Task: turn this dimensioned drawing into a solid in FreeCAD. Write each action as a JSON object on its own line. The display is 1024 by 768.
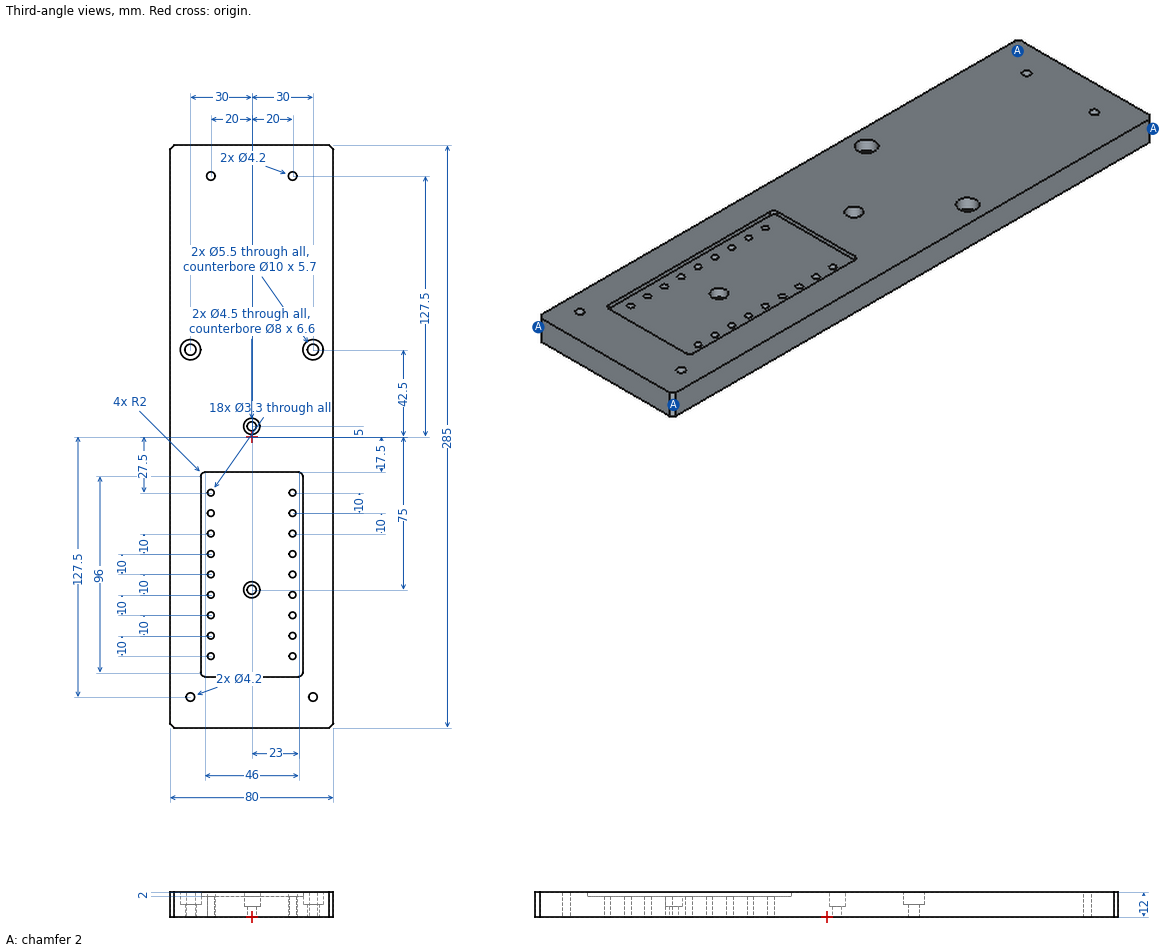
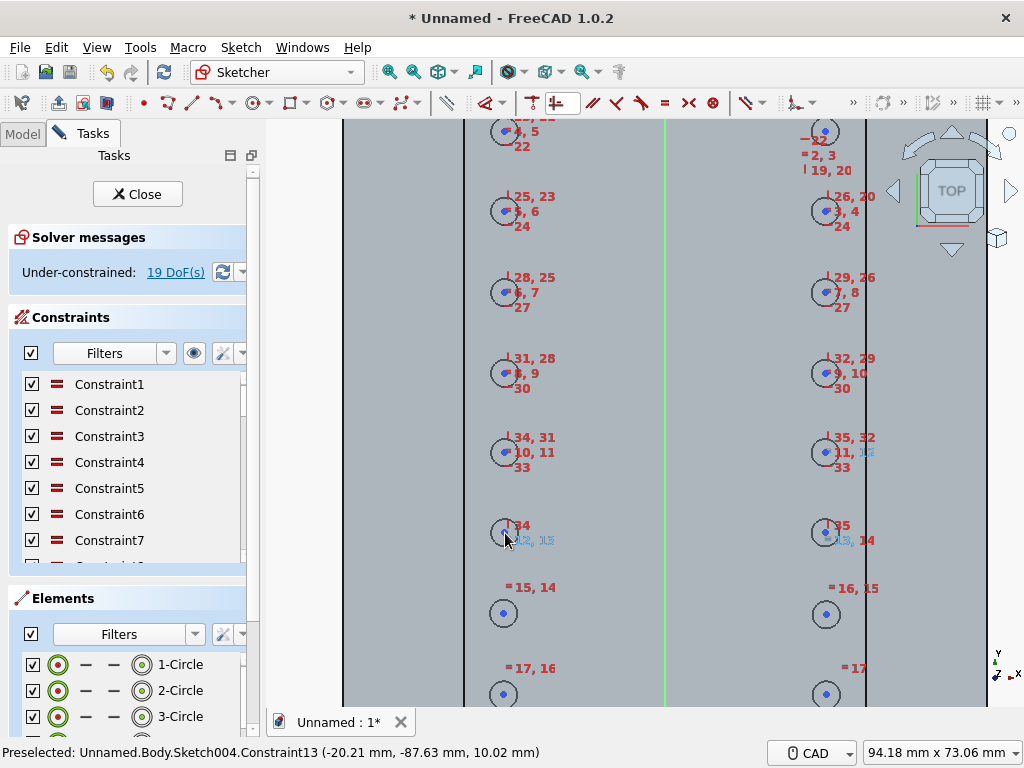
{"action": "scroll", "coordinate": [505, 533], "scroll_direction": "up", "scroll_amount": 4}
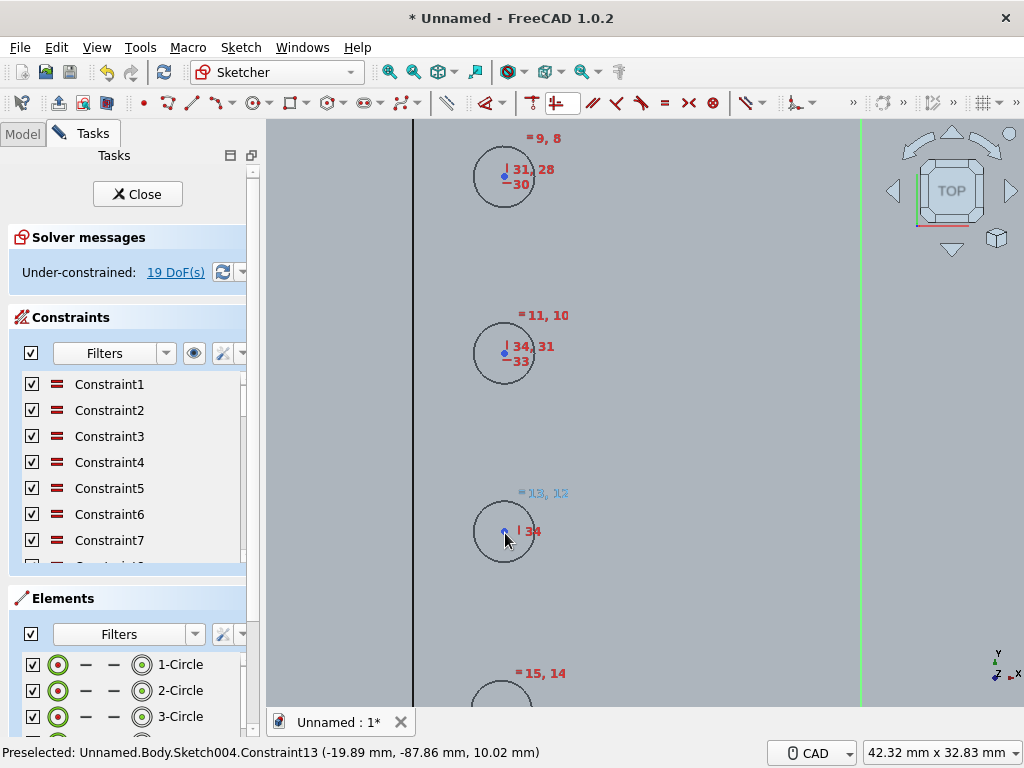
{"action": "left_click", "coordinate": [504, 532]}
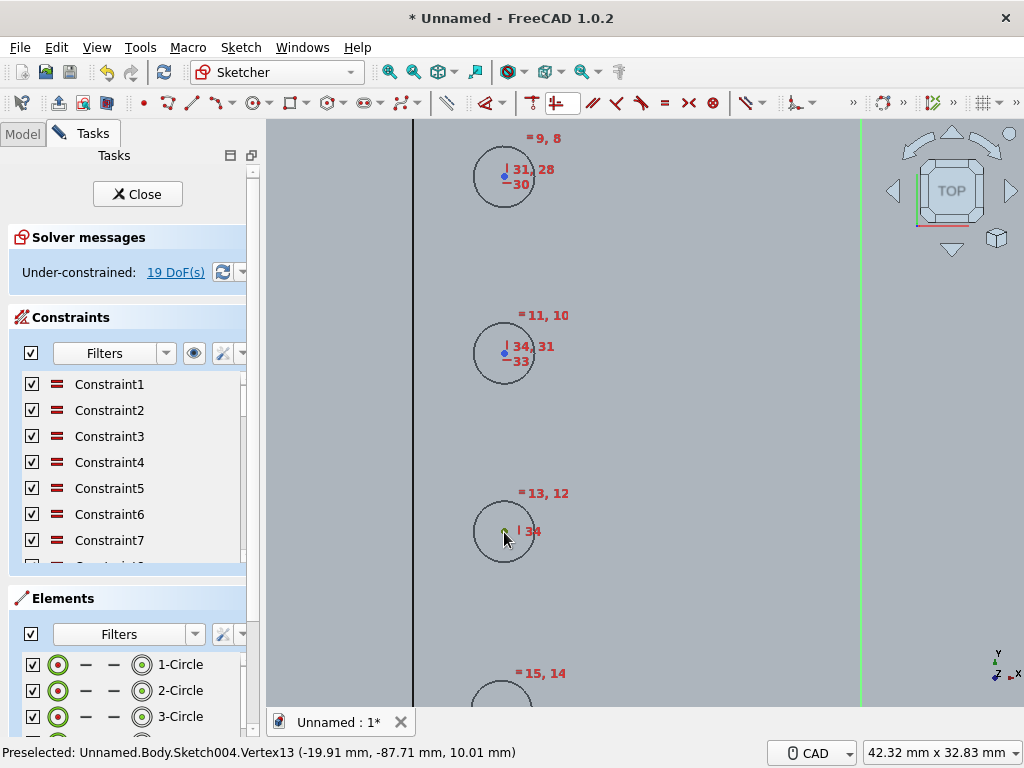
{"action": "scroll", "coordinate": [505, 533], "scroll_direction": "down", "scroll_amount": 8}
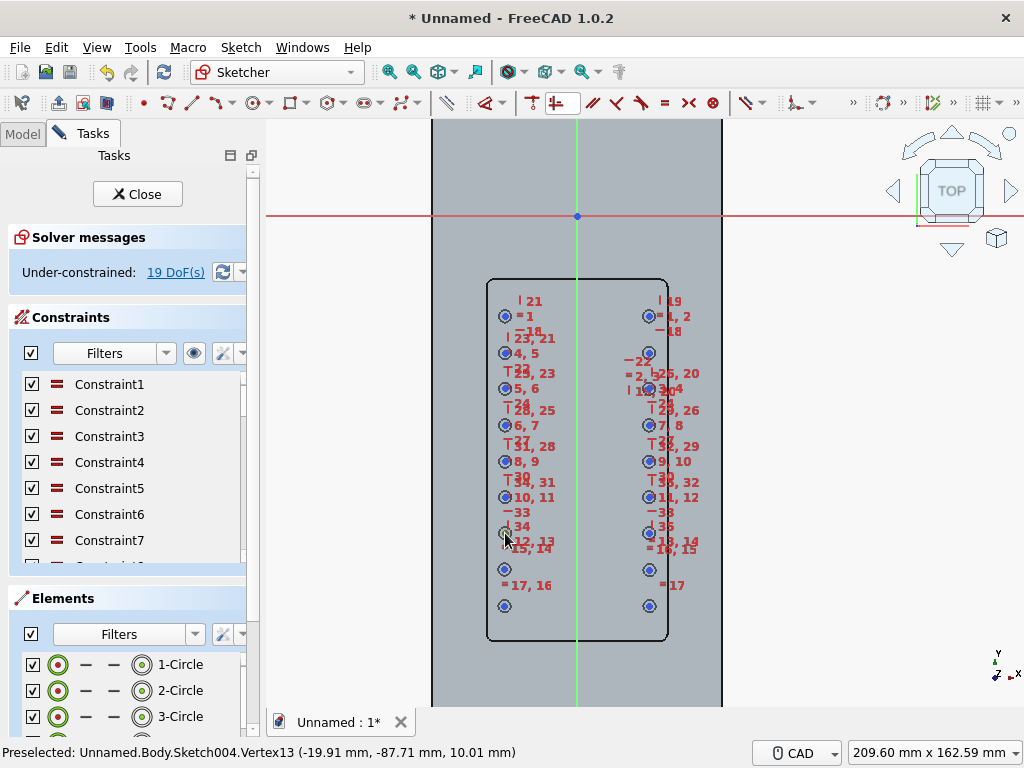
{"action": "scroll", "coordinate": [649, 533], "scroll_direction": "up", "scroll_amount": 4}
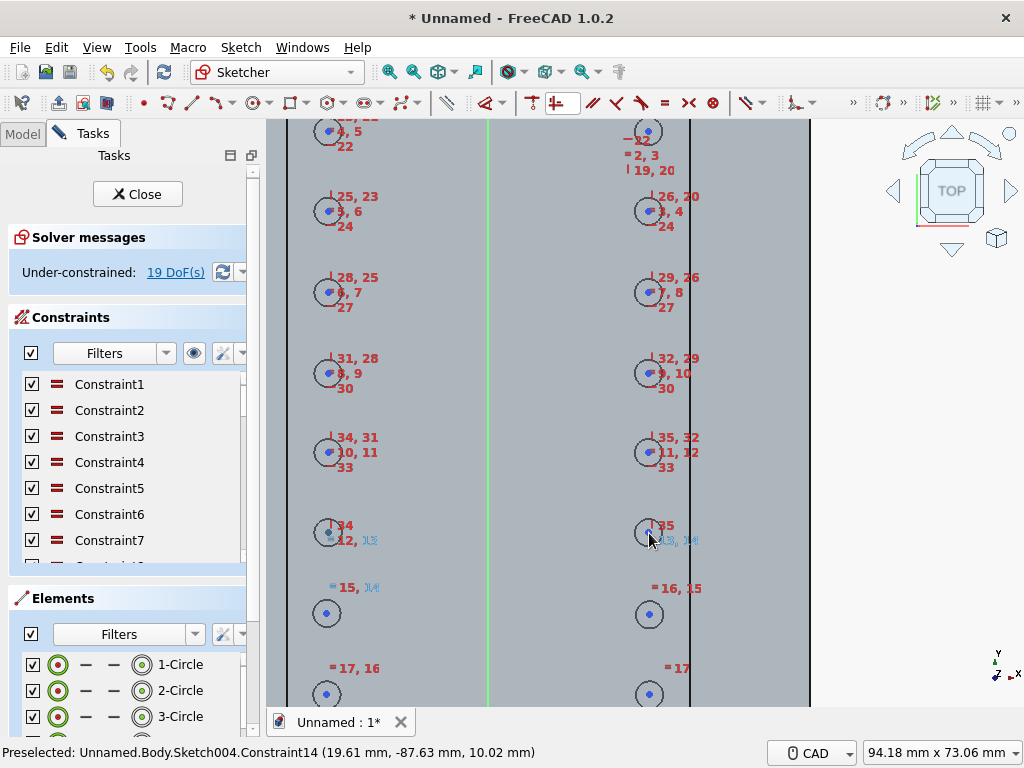
{"action": "scroll", "coordinate": [649, 533], "scroll_direction": "up", "scroll_amount": 4}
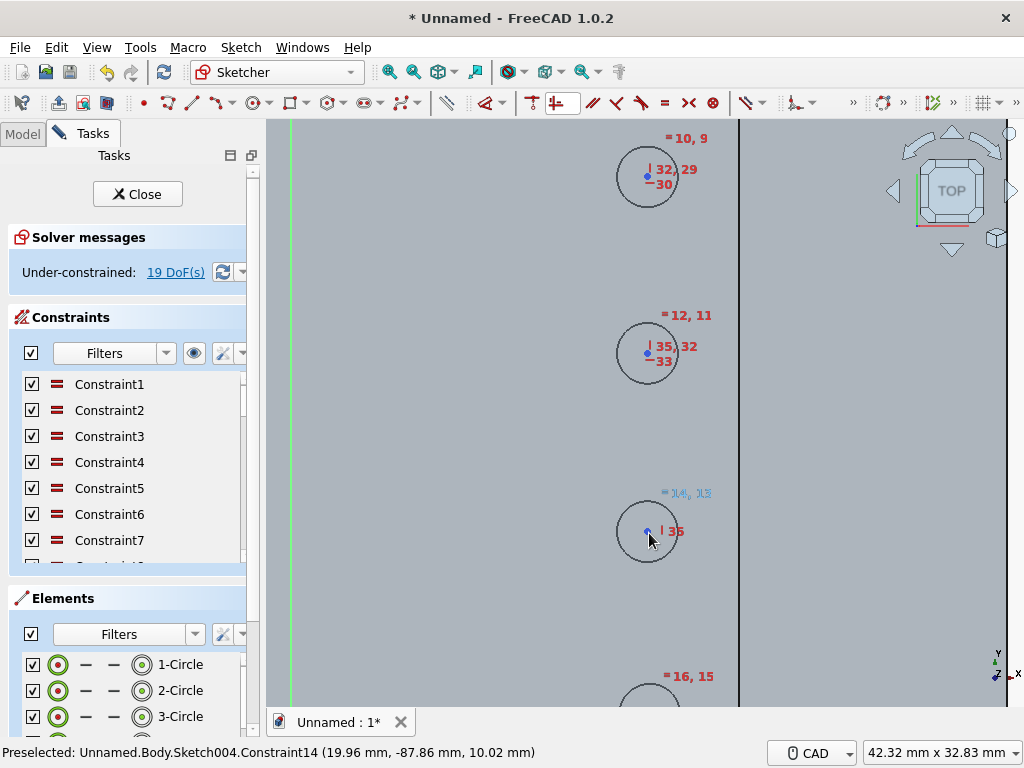
{"action": "left_click", "coordinate": [647, 532]}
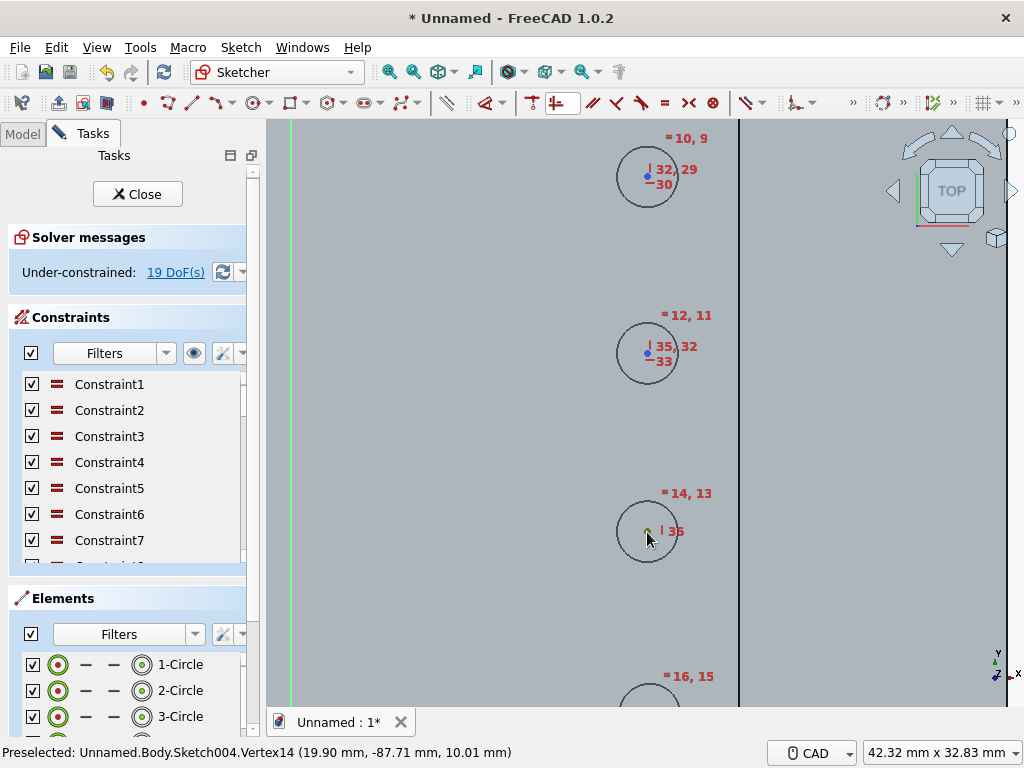
{"action": "key", "text": "h"}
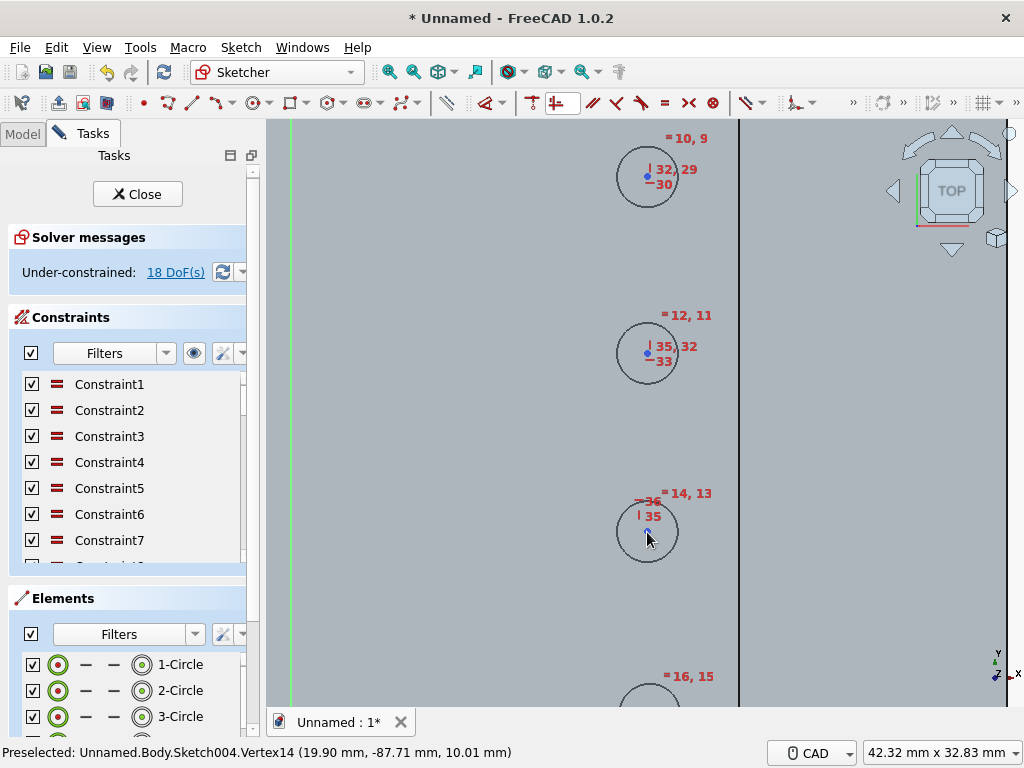
{"action": "scroll", "coordinate": [649, 533], "scroll_direction": "down", "scroll_amount": 8}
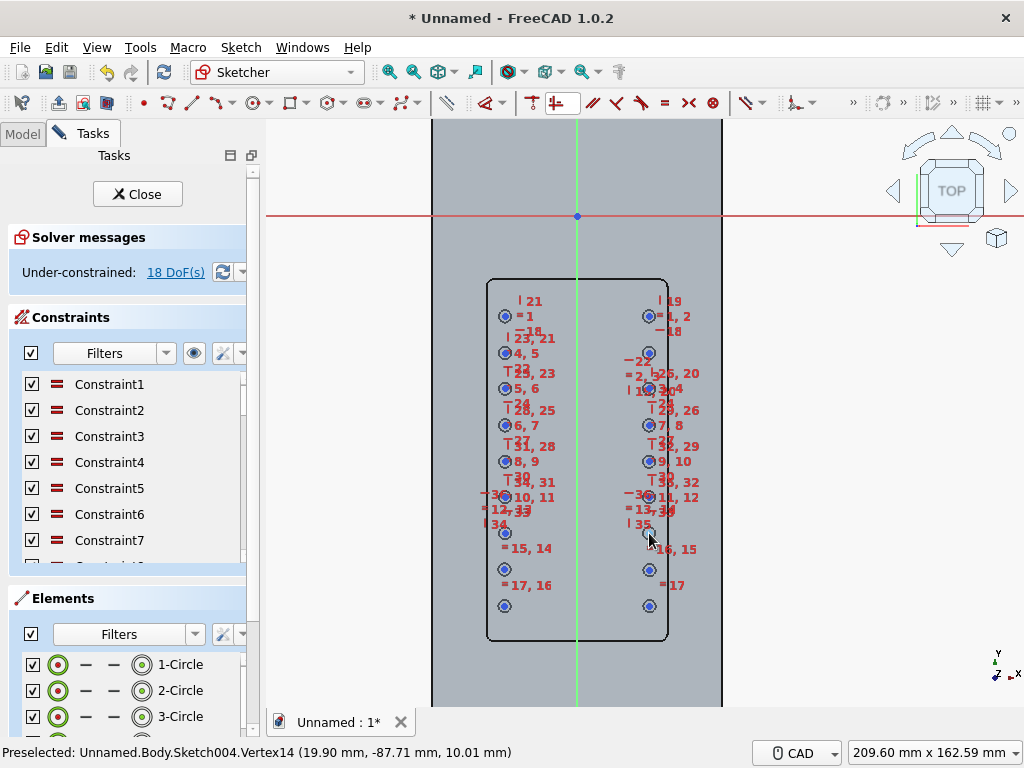
{"action": "left_click", "coordinate": [505, 533]}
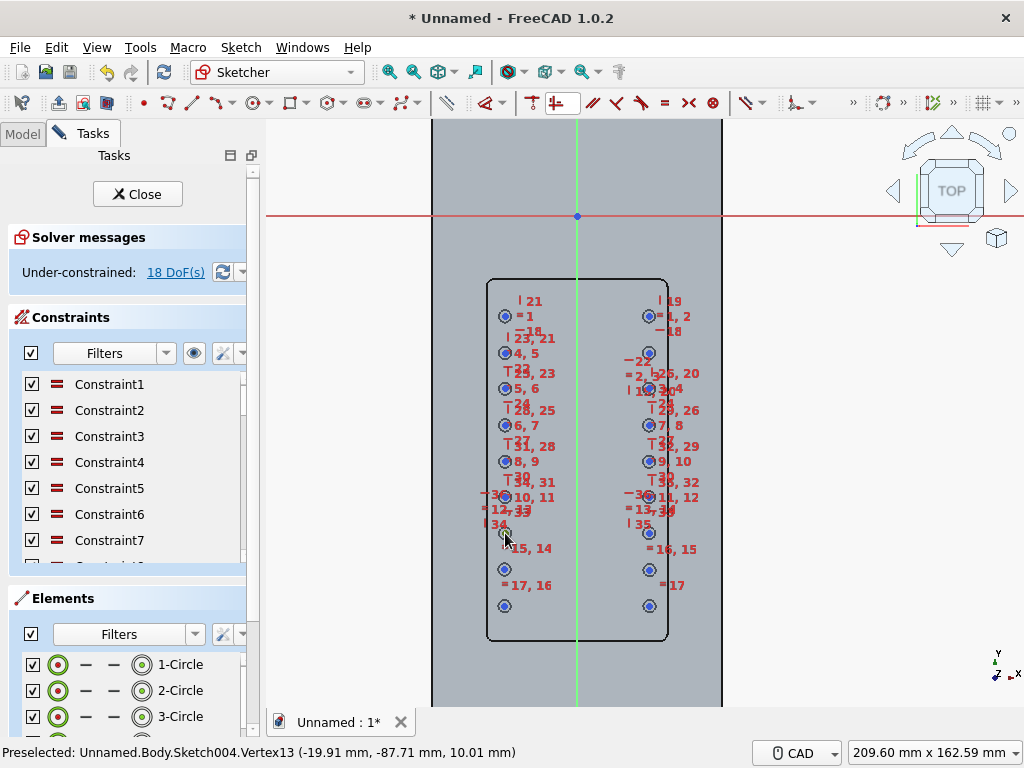
{"action": "left_click", "coordinate": [505, 570]}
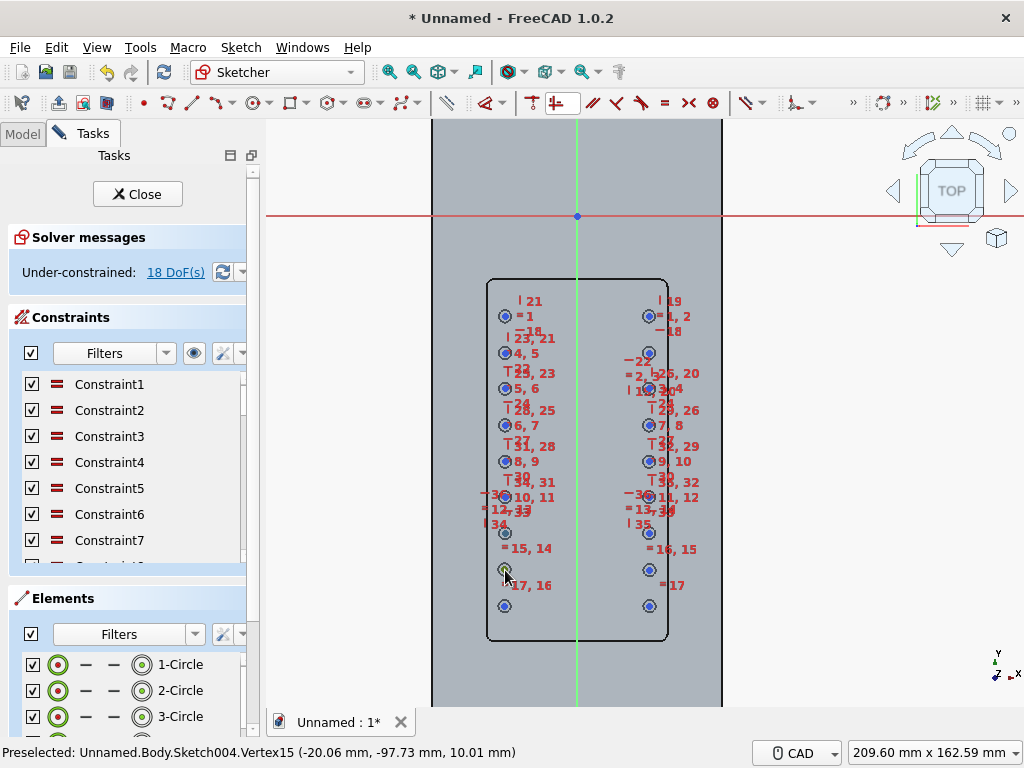
{"action": "key", "text": "v"}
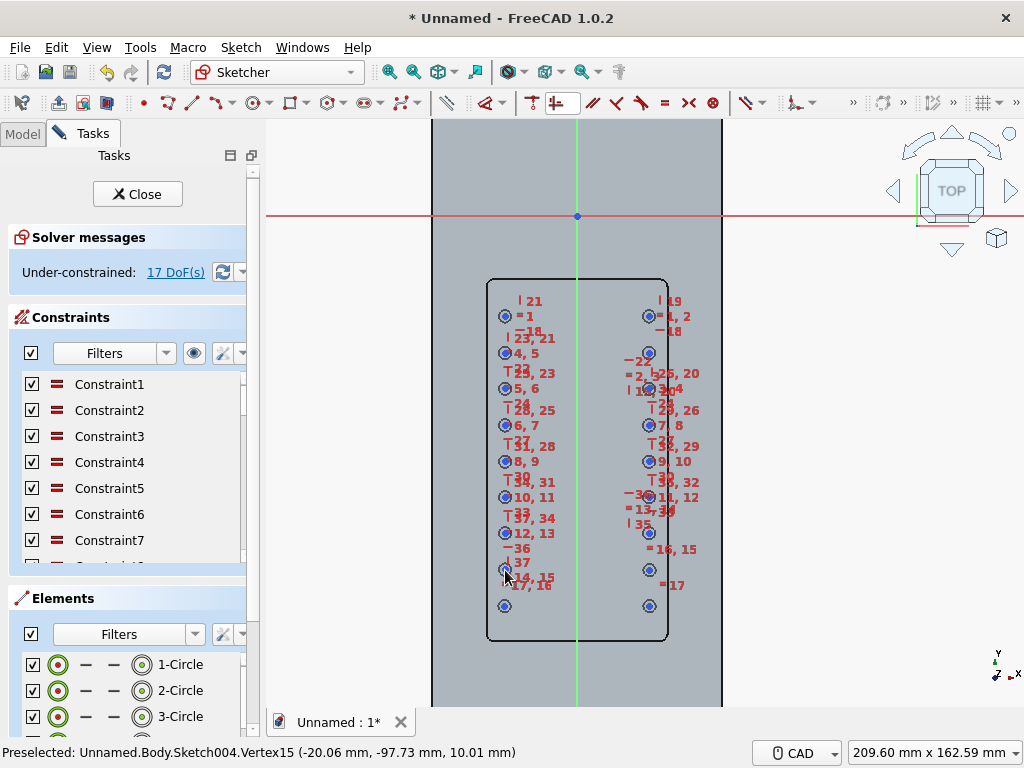
{"action": "left_click", "coordinate": [649, 533]}